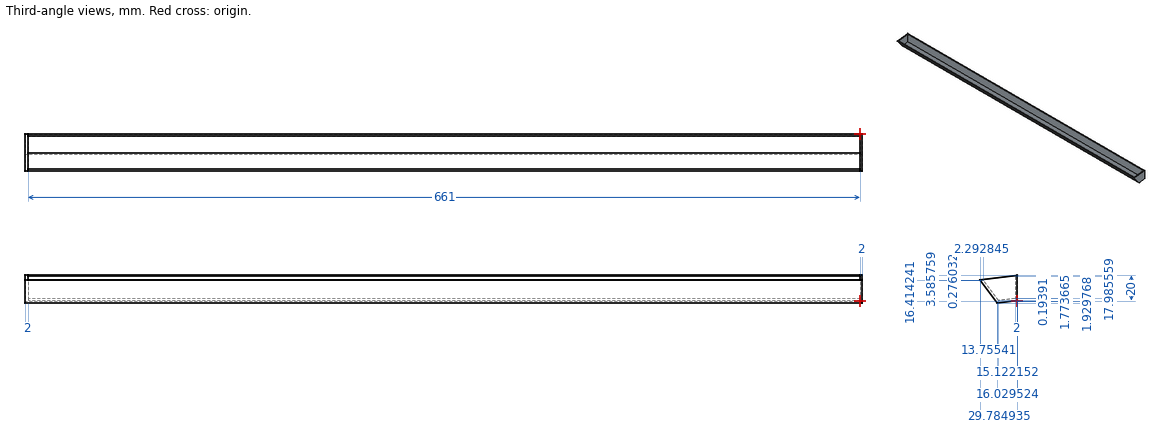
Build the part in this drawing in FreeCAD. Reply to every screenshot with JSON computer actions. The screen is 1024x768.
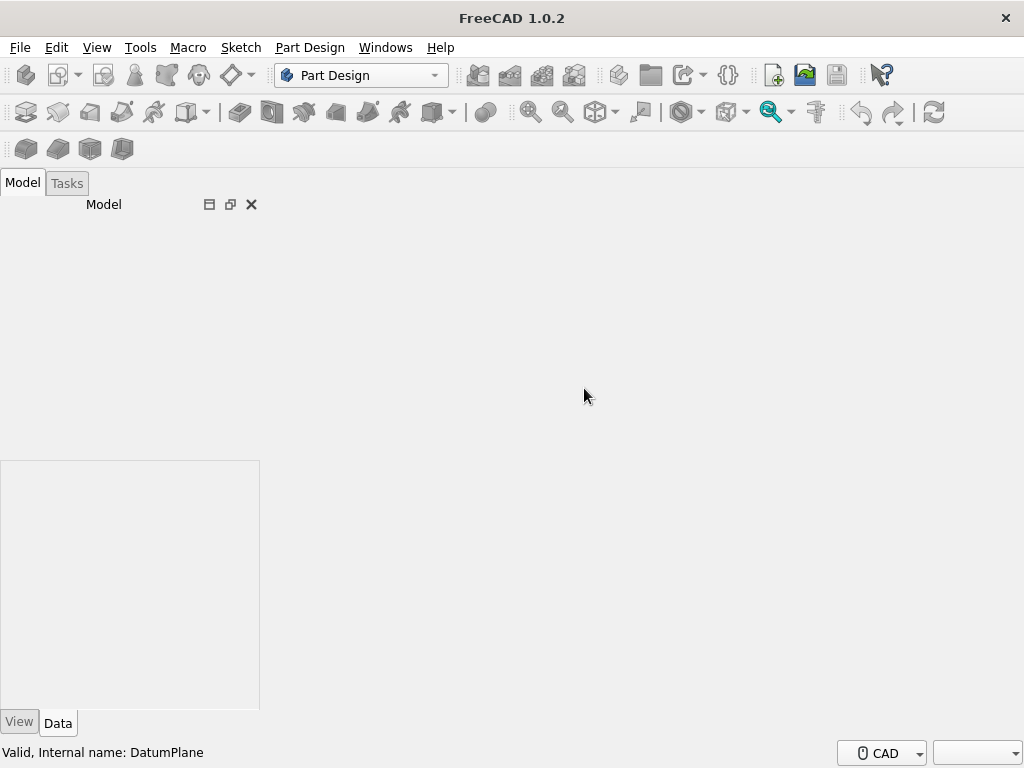
{"action": "key", "text": "ctrl+n"}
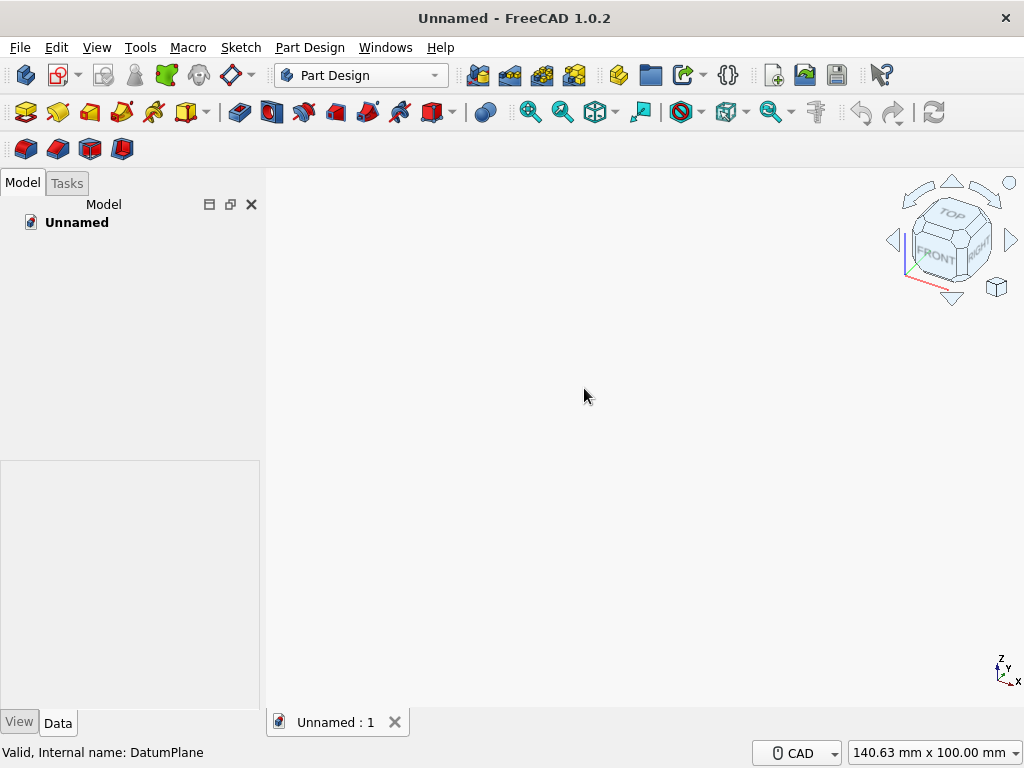
{"action": "left_click", "coordinate": [58, 76]}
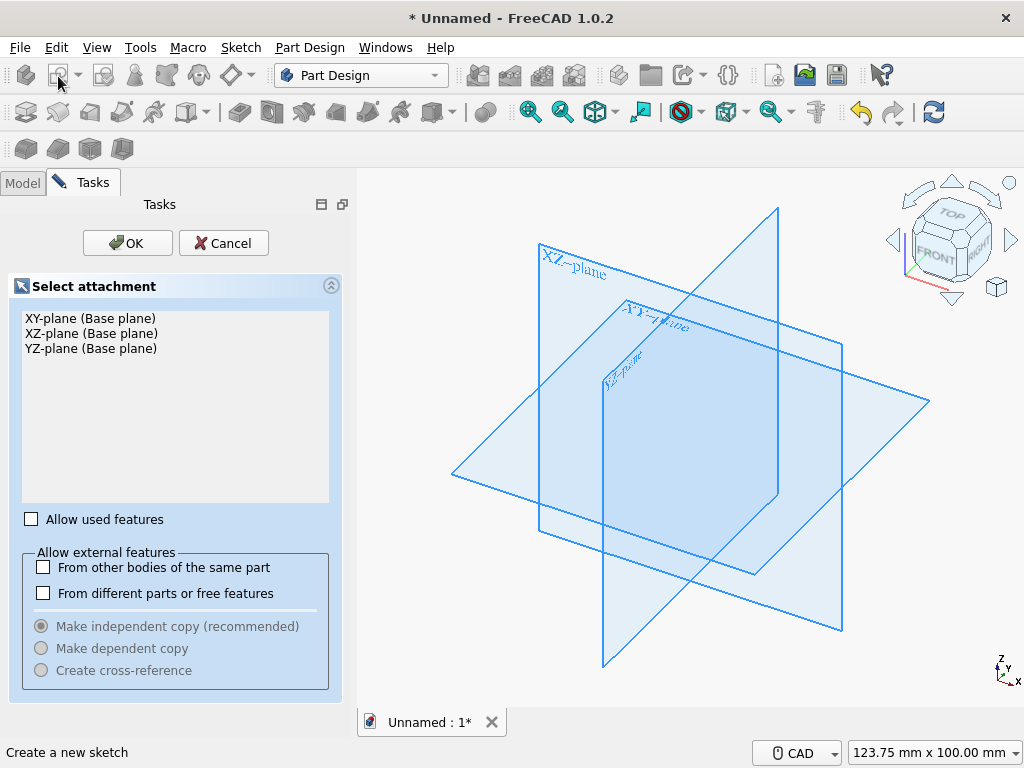
{"action": "left_click", "coordinate": [82, 348]}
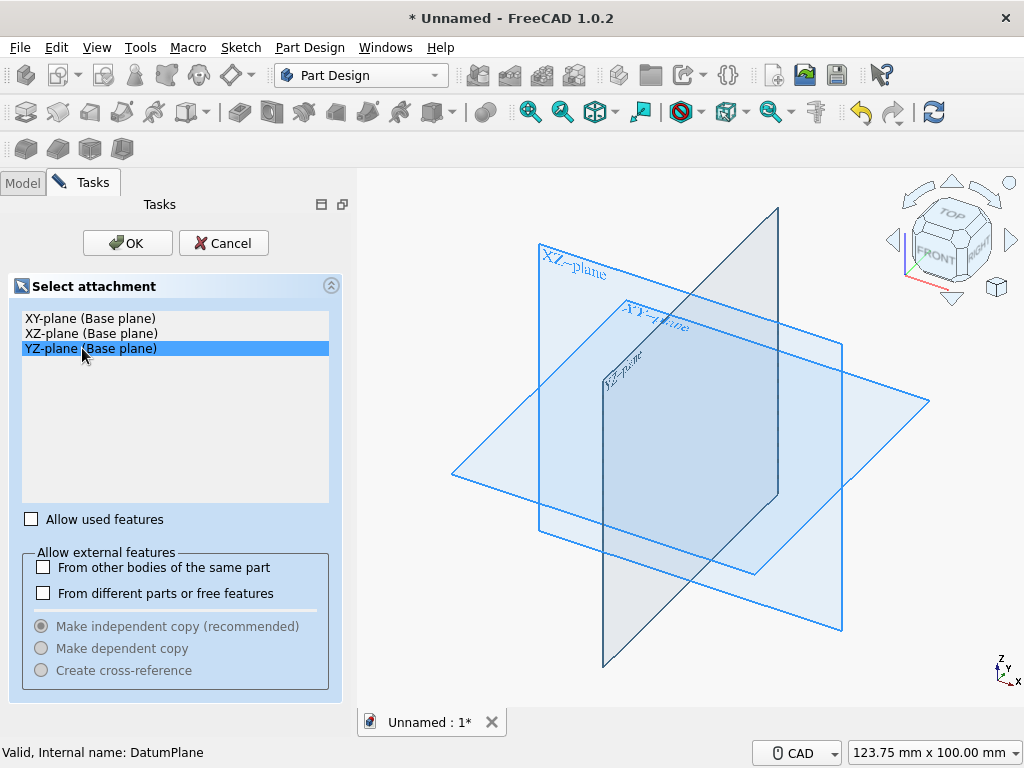
{"action": "left_click", "coordinate": [128, 243]}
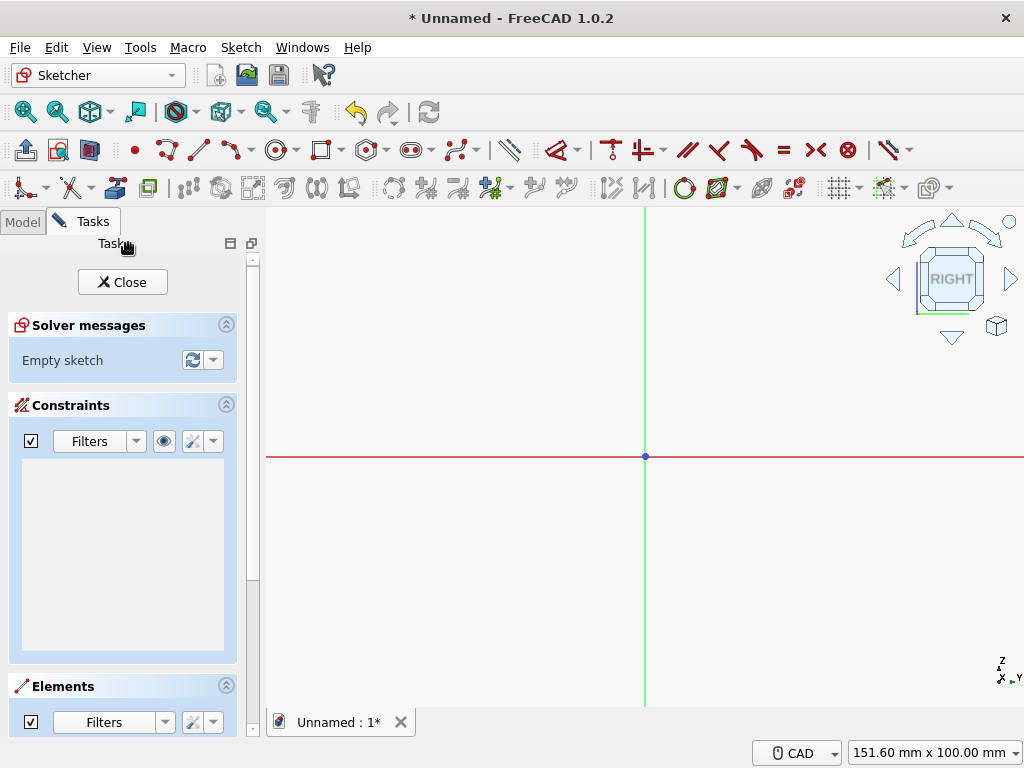
{"action": "scroll", "coordinate": [567, 386], "scroll_direction": "up", "scroll_amount": 5}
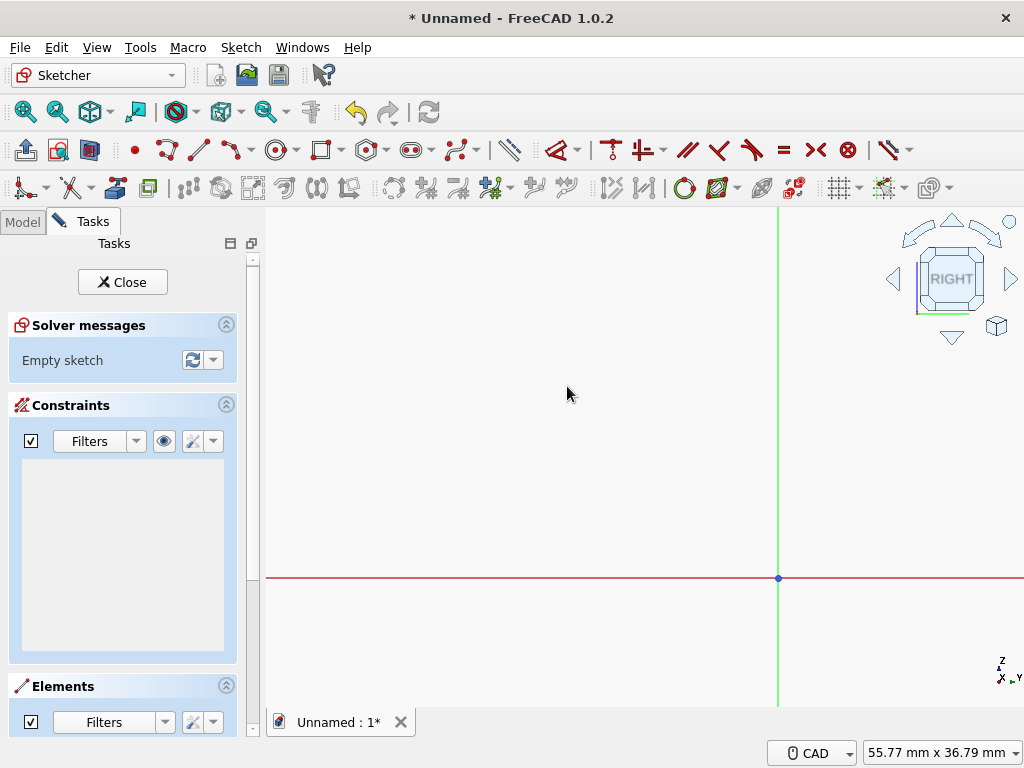
{"action": "left_click", "coordinate": [168, 150]}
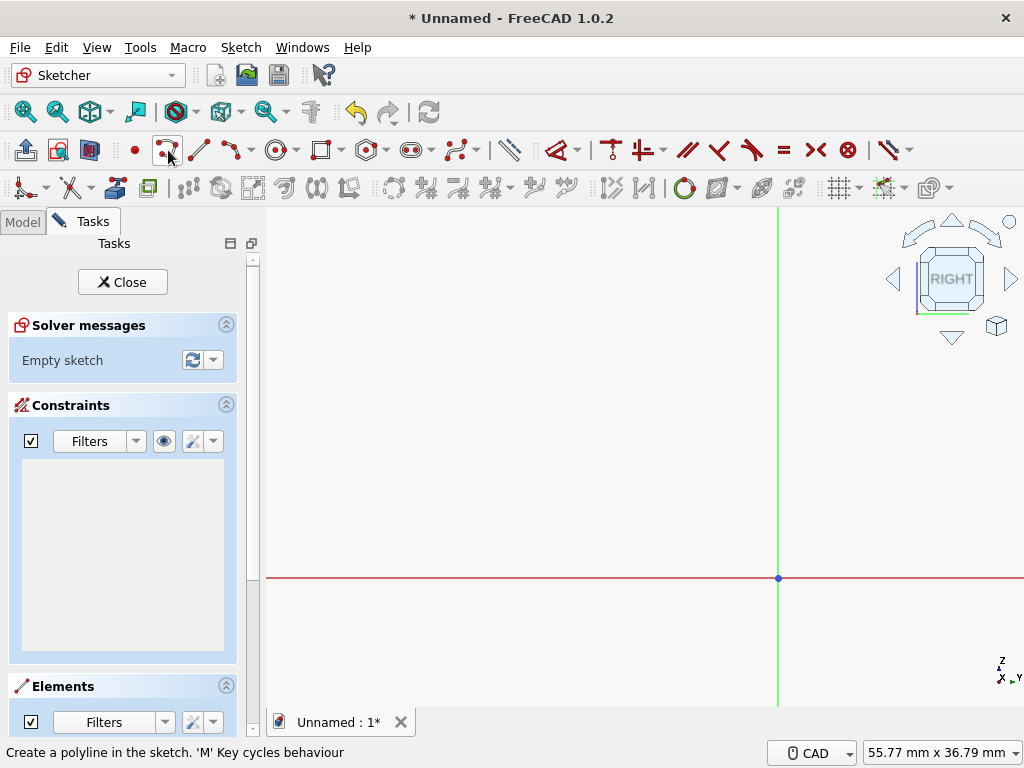
{"action": "left_click", "coordinate": [778, 578]}
{"action": "left_click", "coordinate": [769, 307]}
{"action": "left_click", "coordinate": [374, 355]}
{"action": "left_click", "coordinate": [560, 605]}
{"action": "left_click", "coordinate": [778, 578]}
{"action": "key", "text": "Escape"}
{"action": "key", "text": "Escape"}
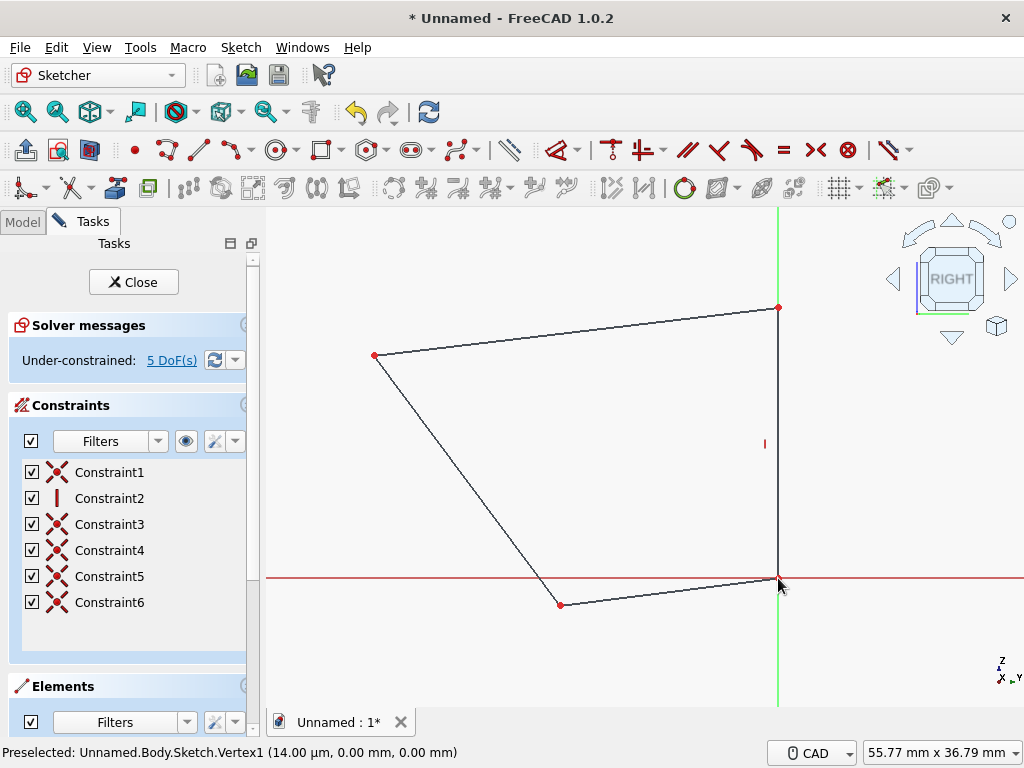
{"action": "key", "text": "d"}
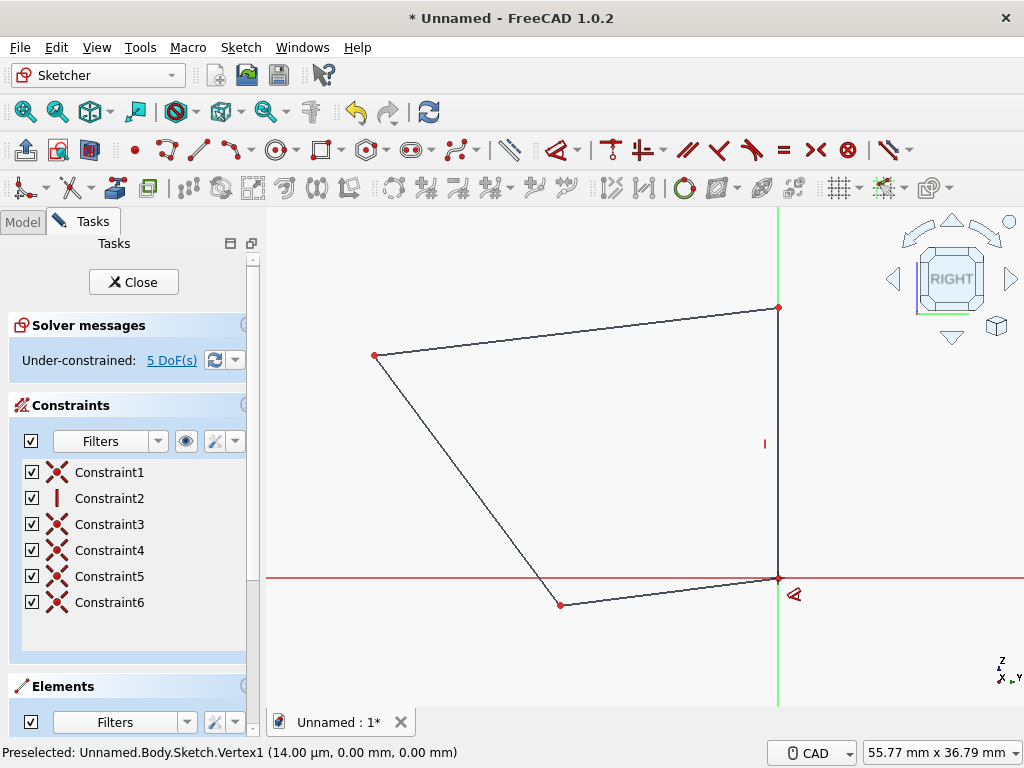
{"action": "left_click", "coordinate": [778, 497]}
{"action": "left_click", "coordinate": [812, 443]}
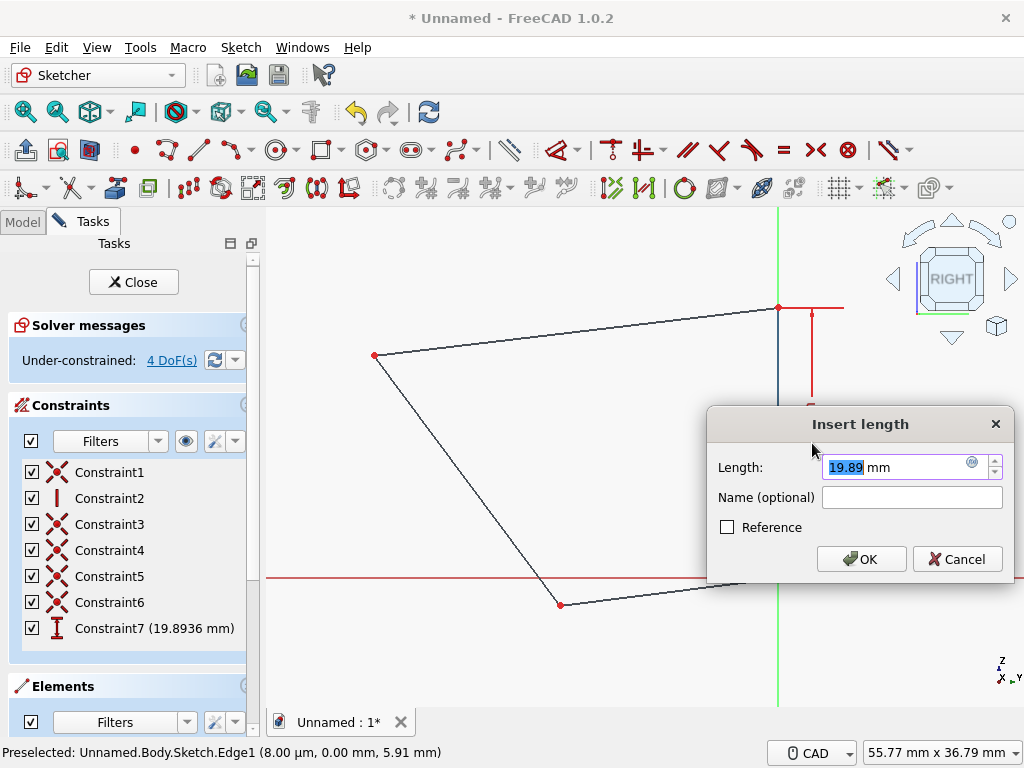
{"action": "type", "text": "20"}
{"action": "key", "text": "Return"}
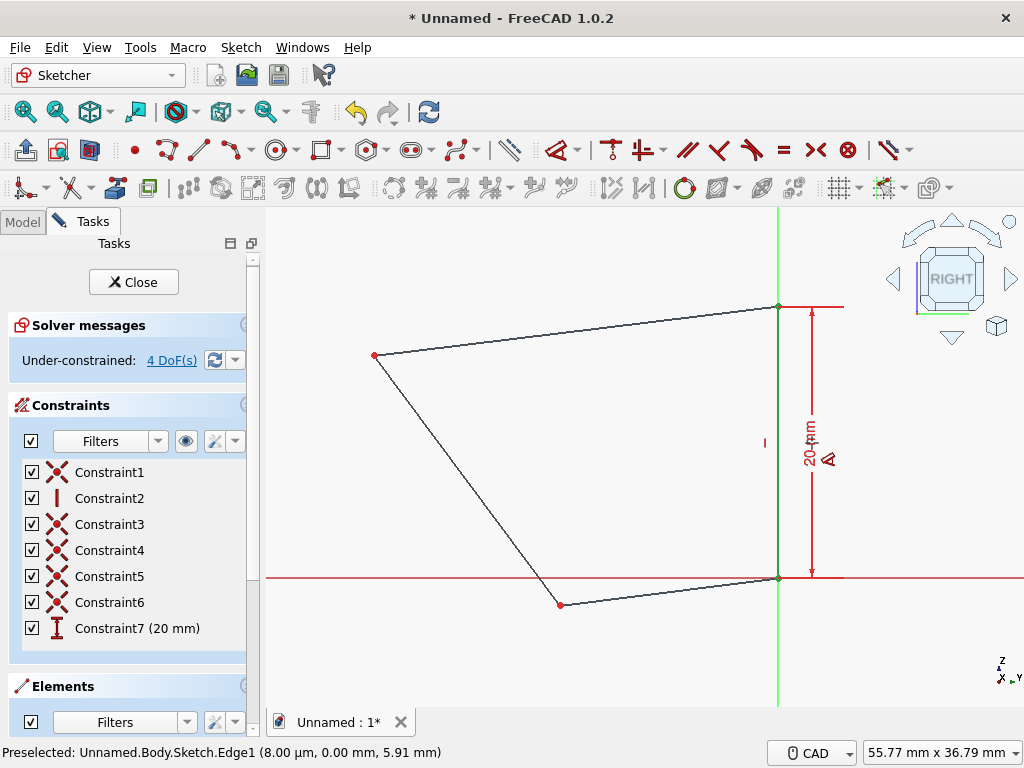
{"action": "scroll", "coordinate": [560, 606], "scroll_direction": "up", "scroll_amount": 3}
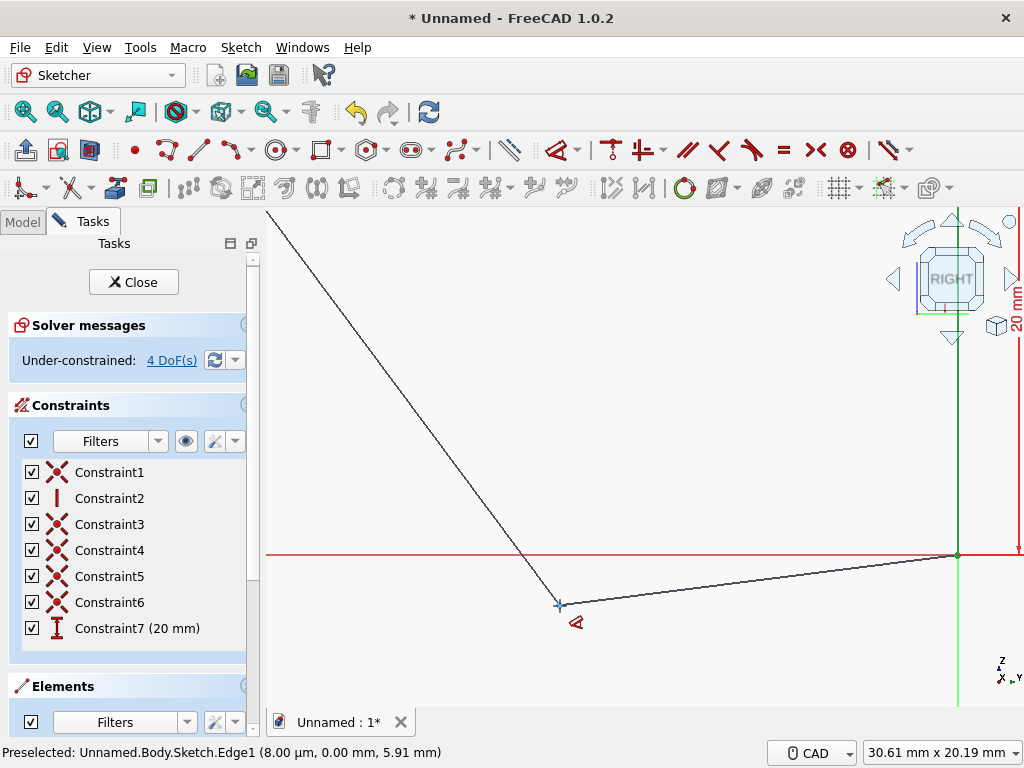
{"action": "left_click", "coordinate": [560, 605]}
{"action": "left_click", "coordinate": [526, 592]}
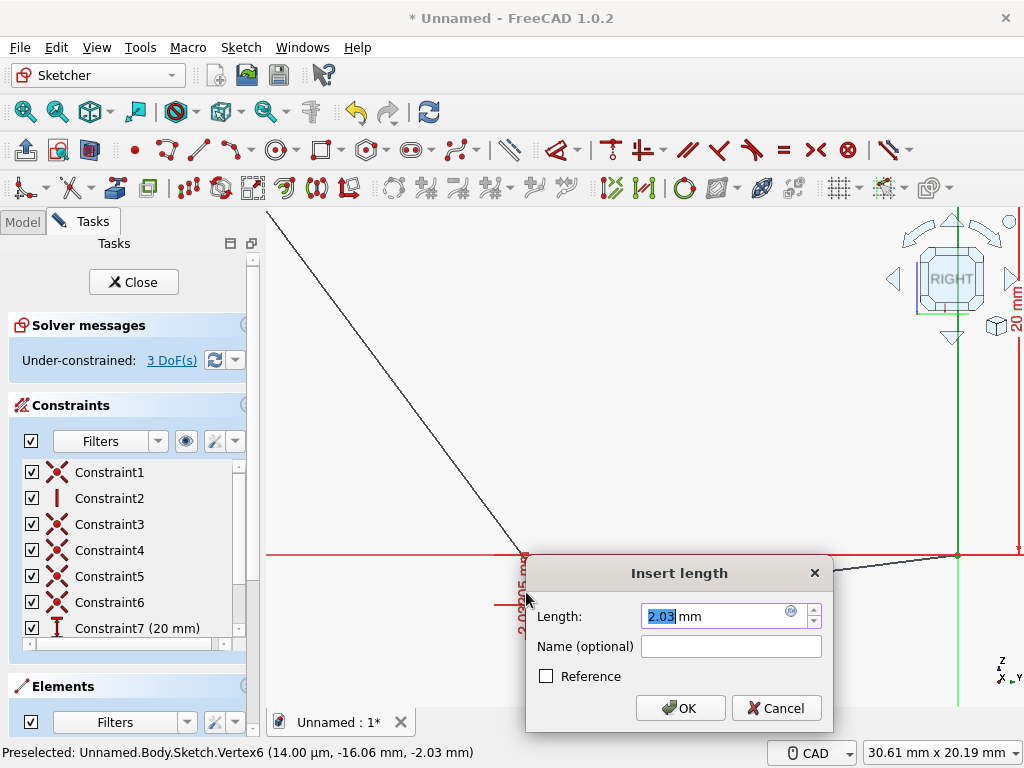
{"action": "type", "text": "1.929768"}
{"action": "key", "text": "Return"}